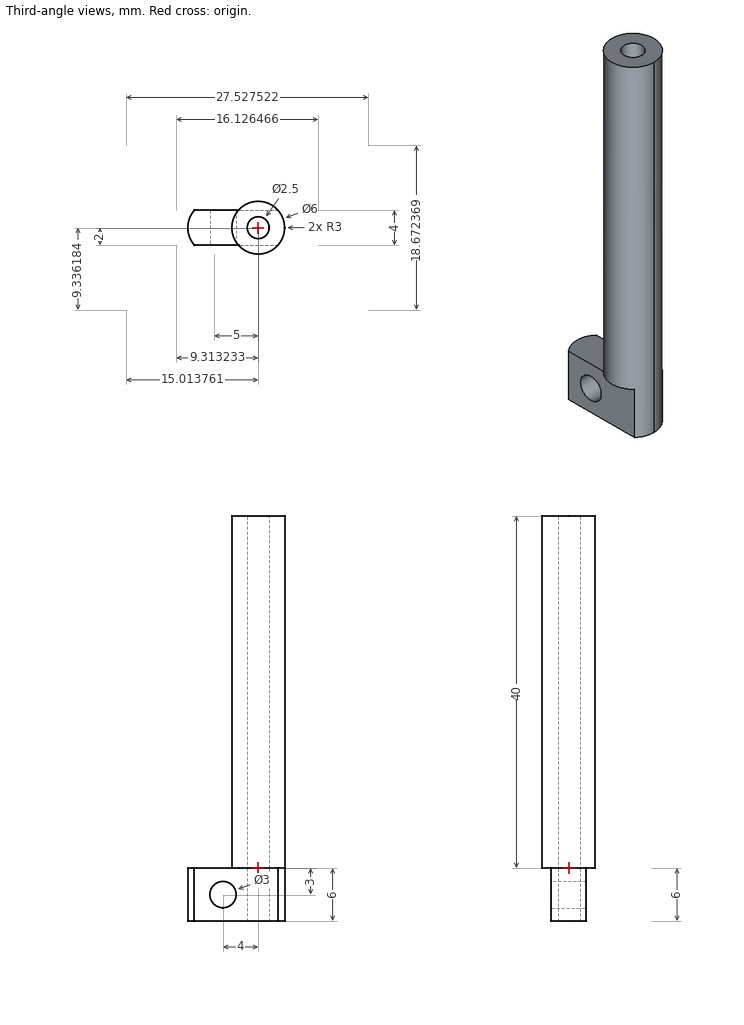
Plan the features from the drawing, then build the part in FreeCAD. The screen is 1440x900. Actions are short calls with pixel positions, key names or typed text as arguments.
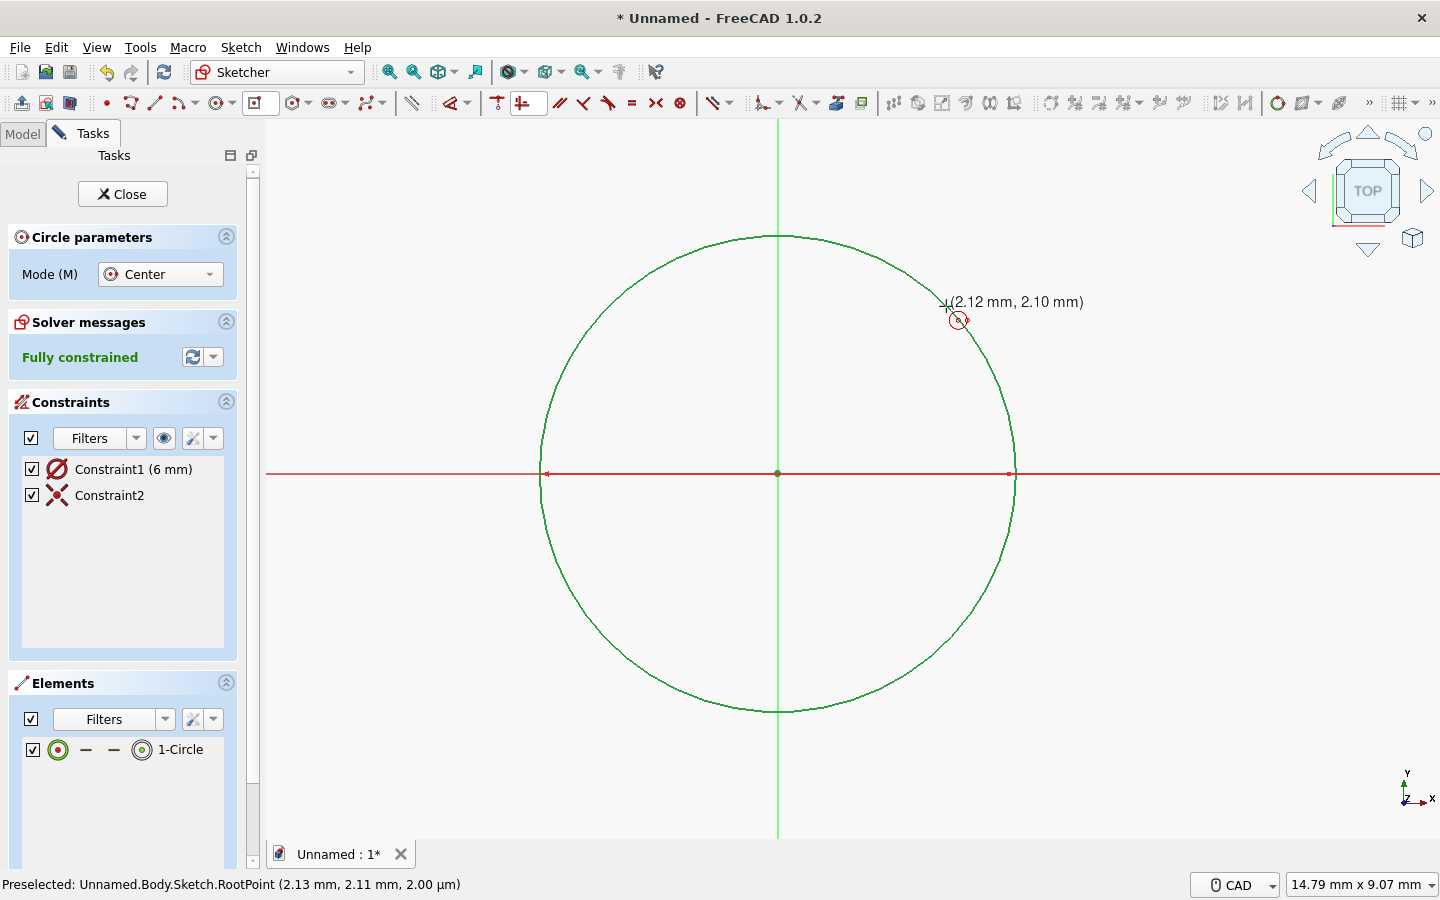
click(778, 474)
move(848, 404)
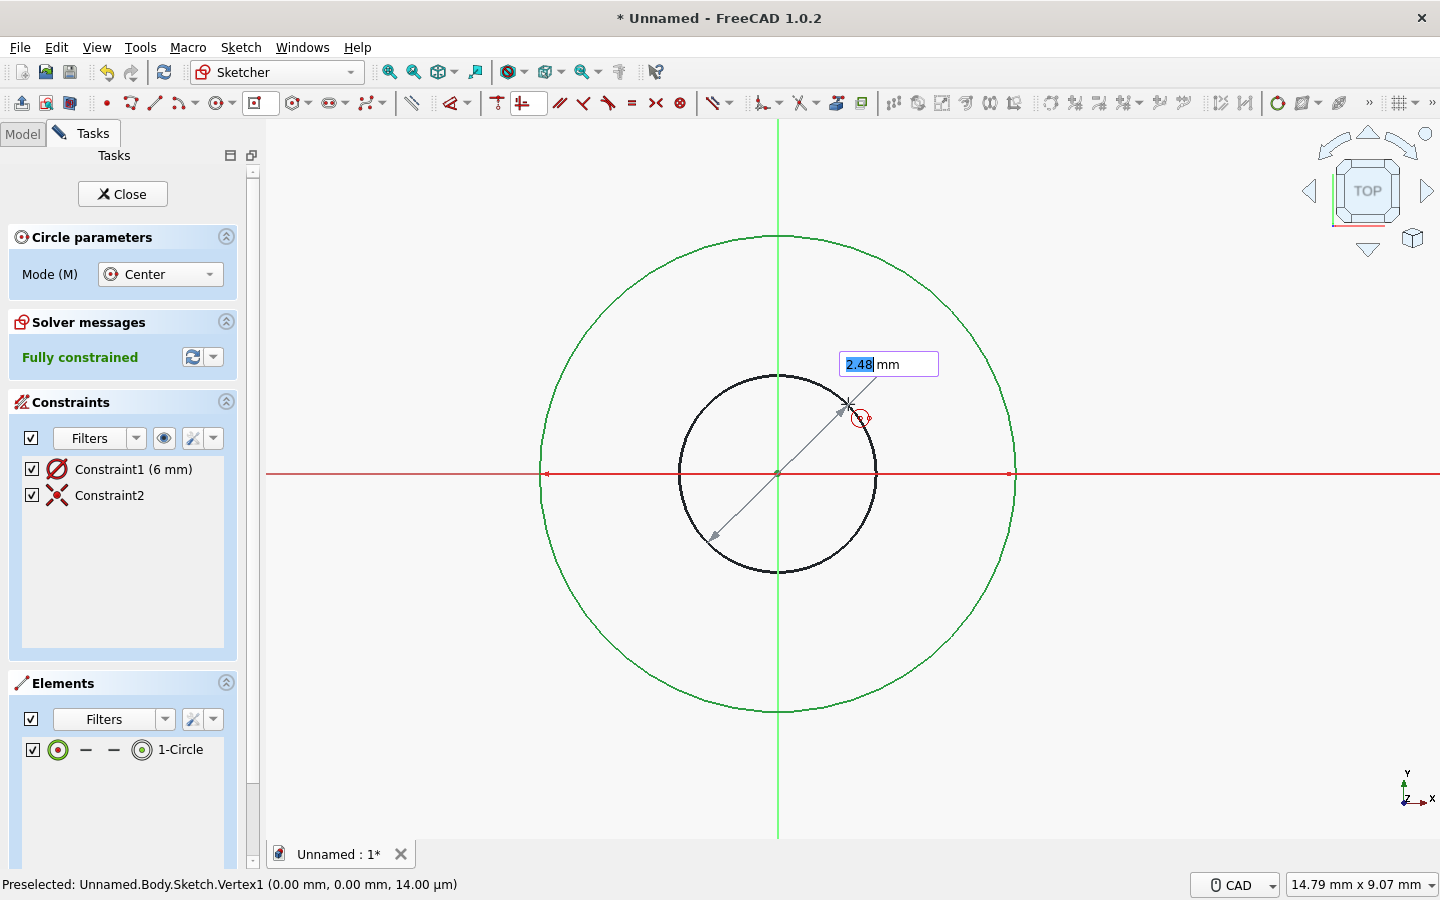
text(2.5)
key(Return)
key(Escape)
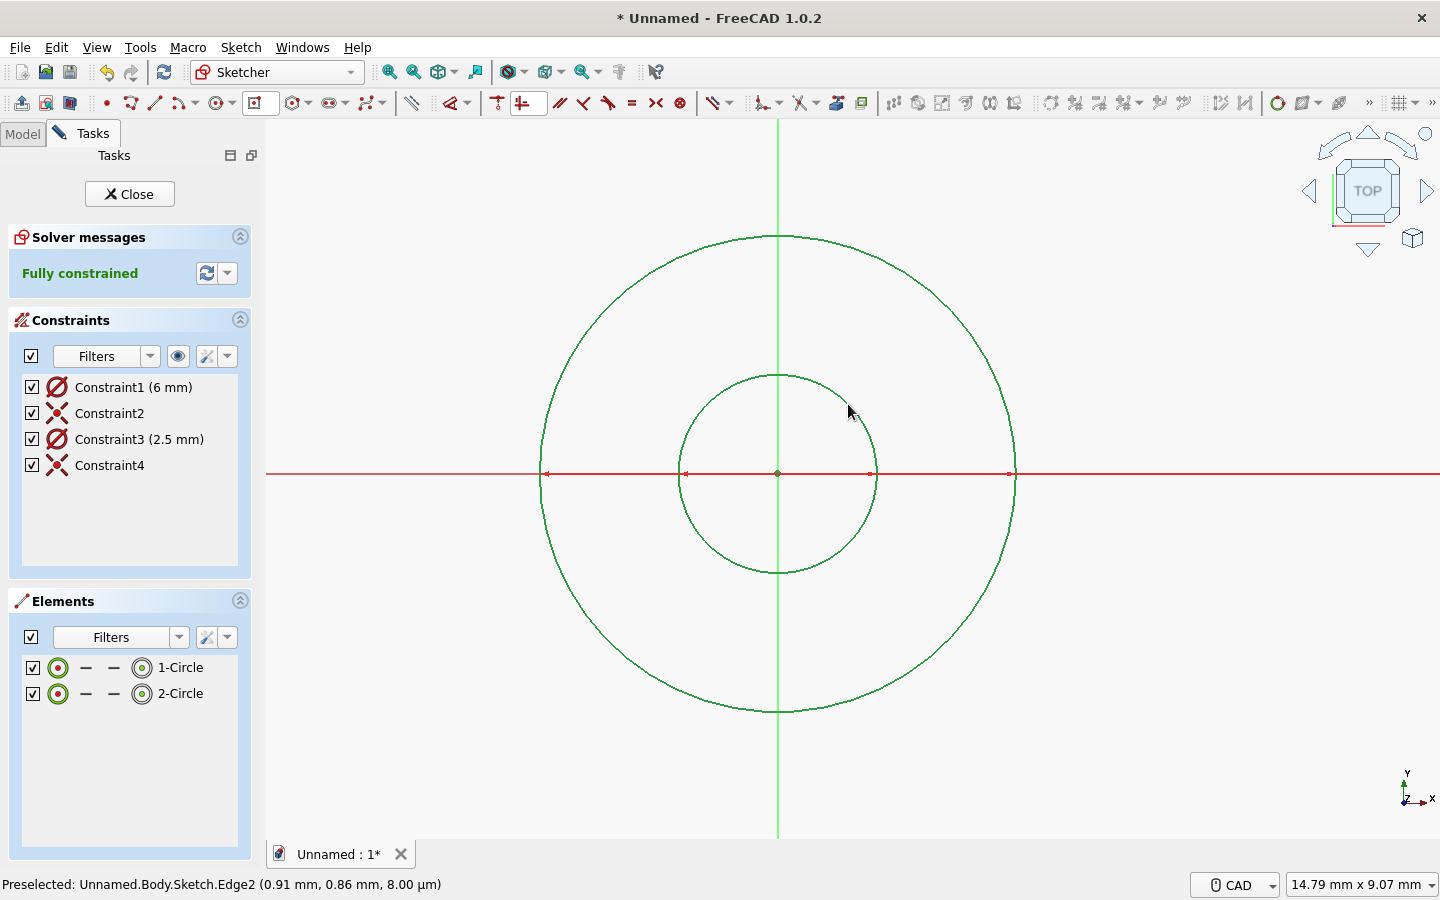
click(130, 194)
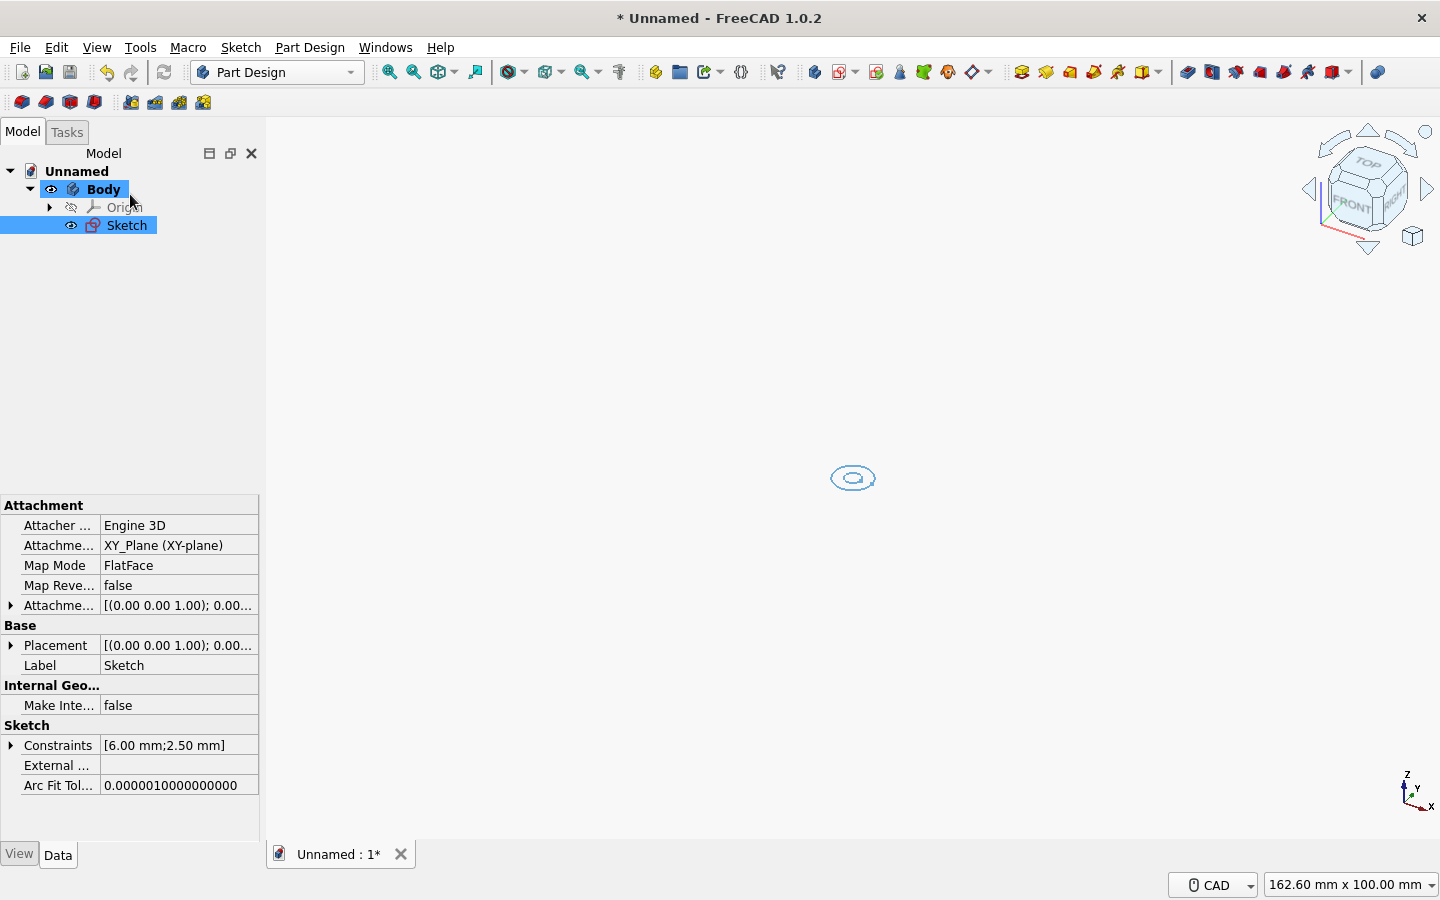
click(1022, 72)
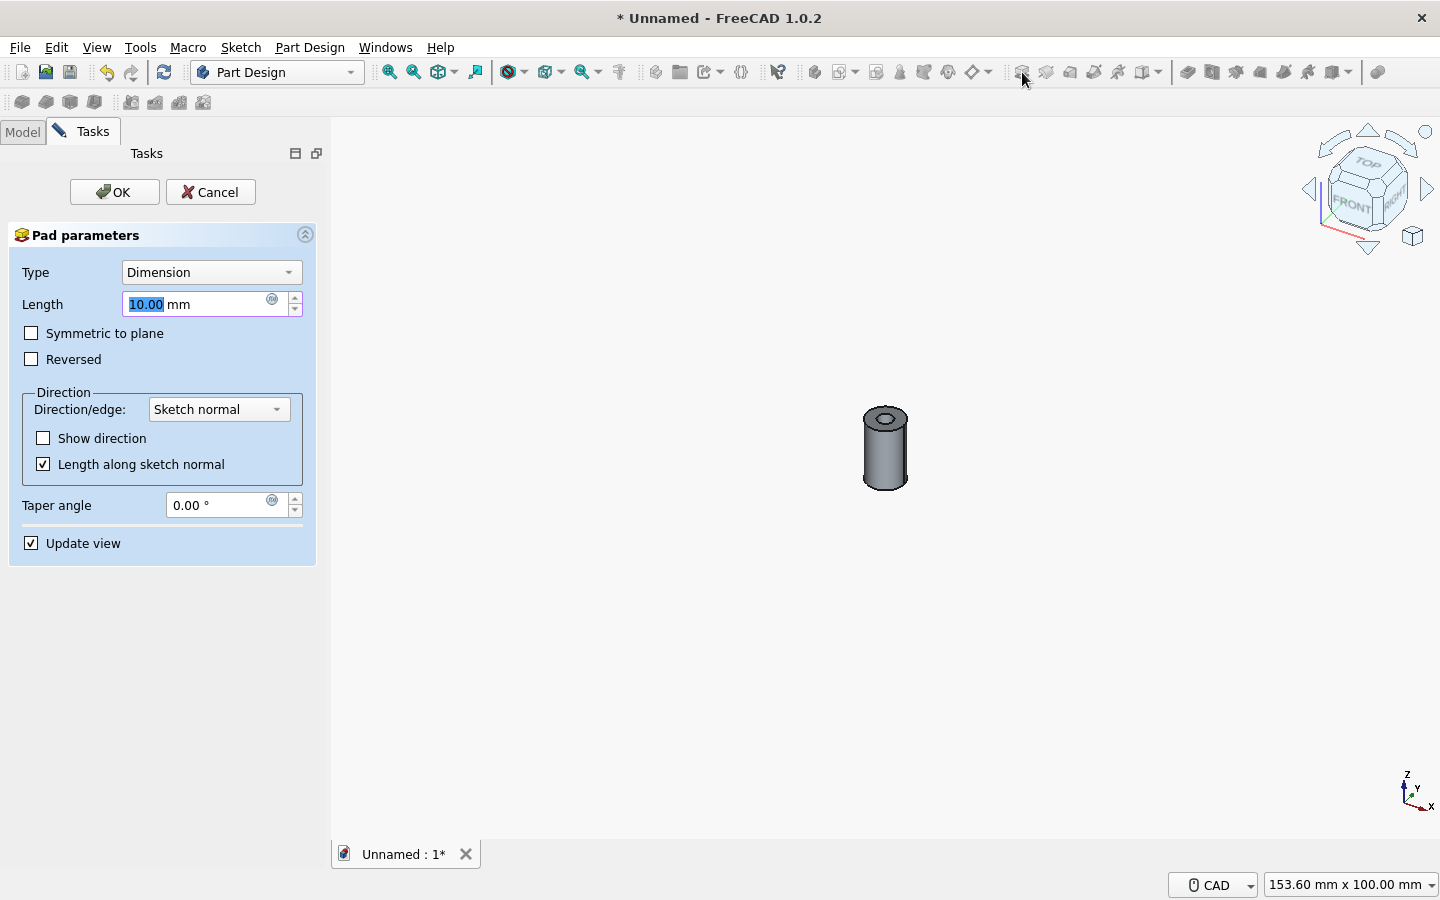
text(40)
key(Tab)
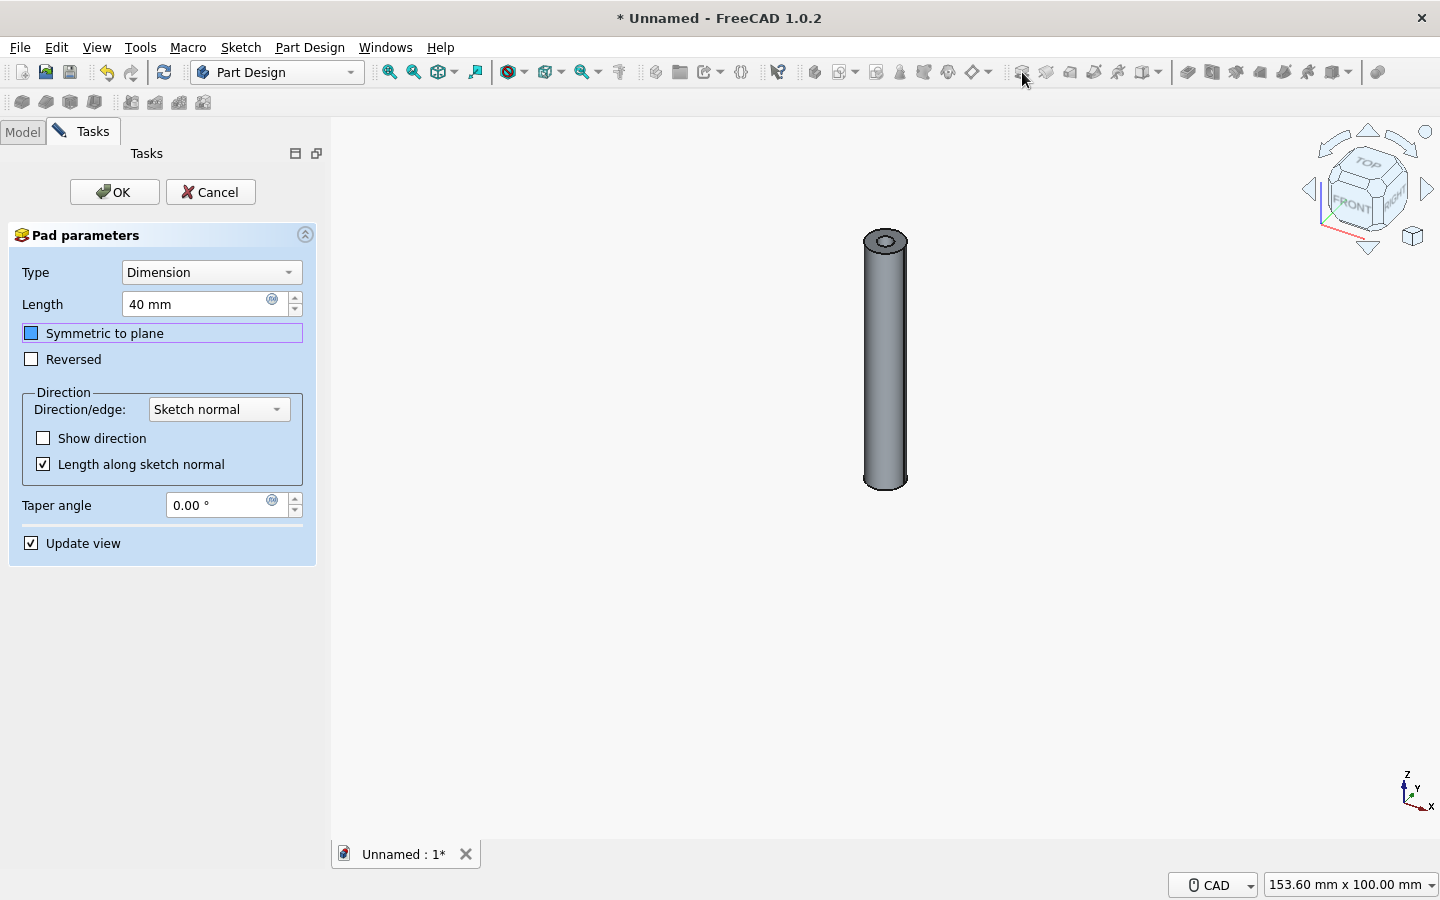
click(115, 192)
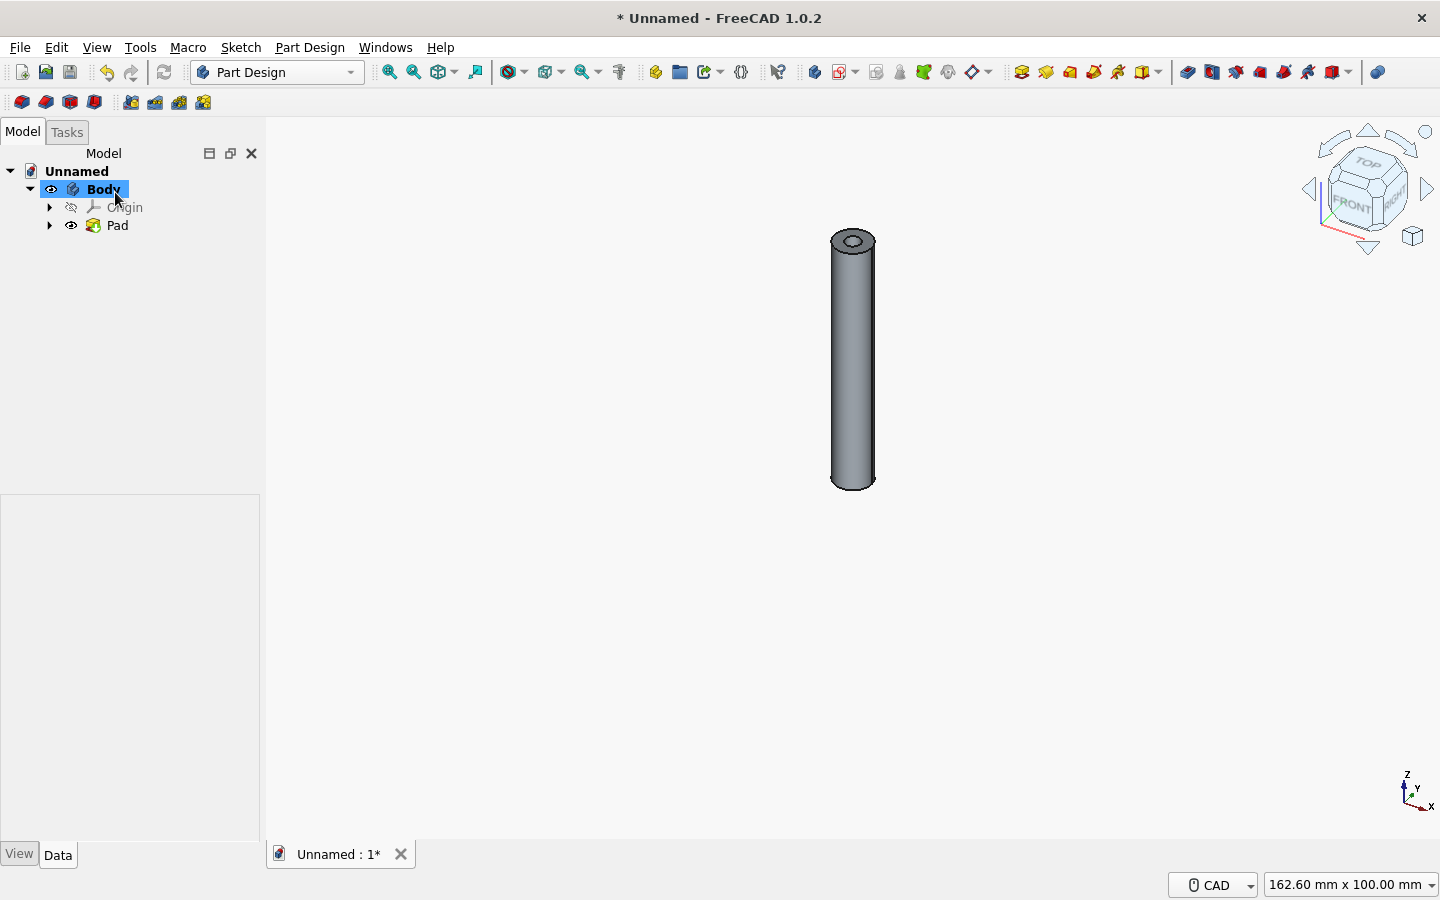
click(390, 72)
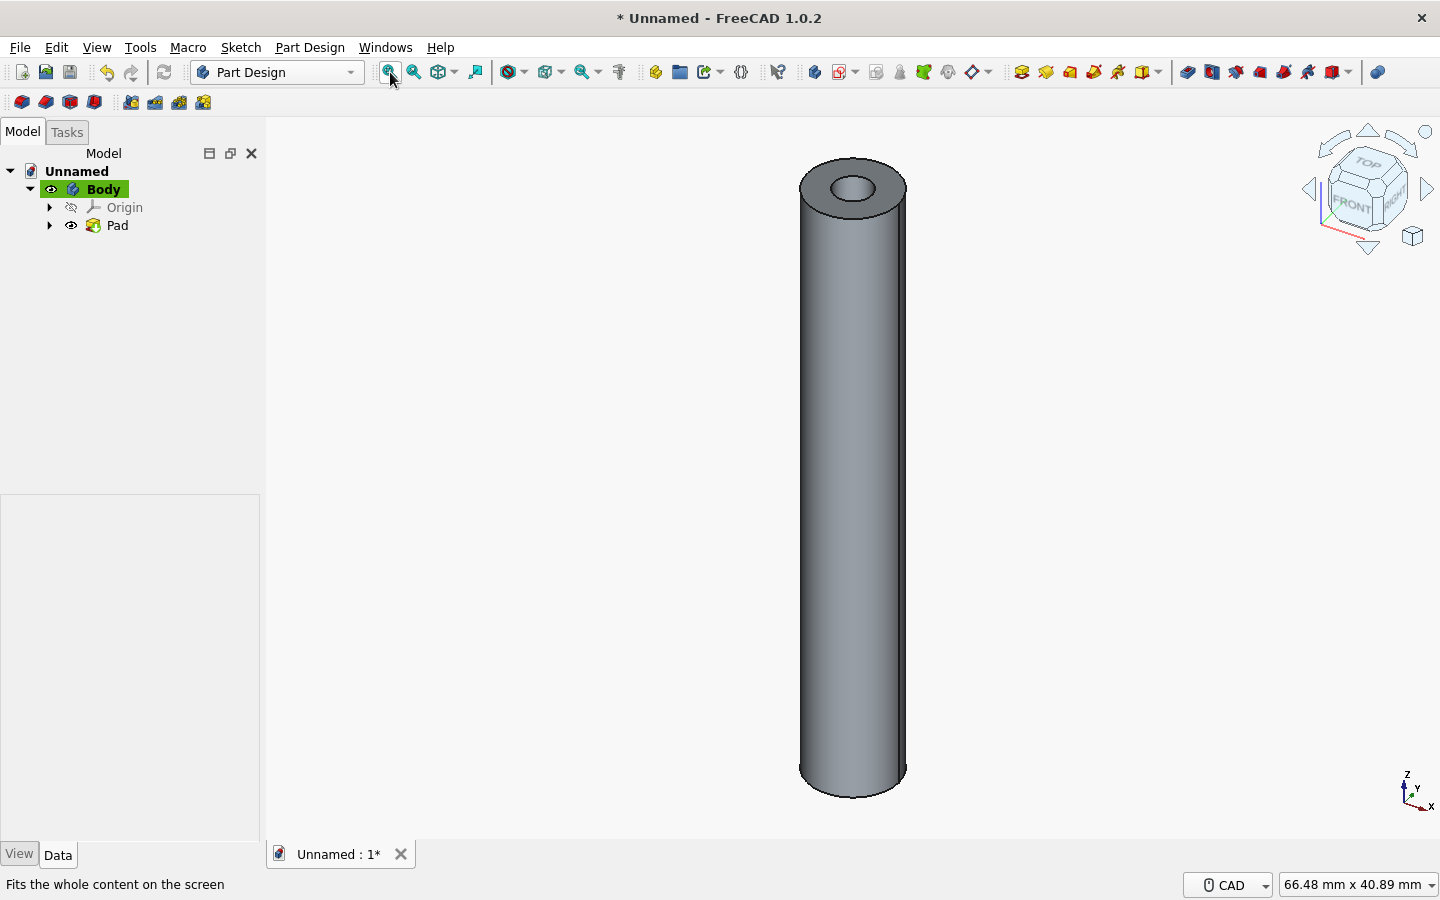
click(50, 207)